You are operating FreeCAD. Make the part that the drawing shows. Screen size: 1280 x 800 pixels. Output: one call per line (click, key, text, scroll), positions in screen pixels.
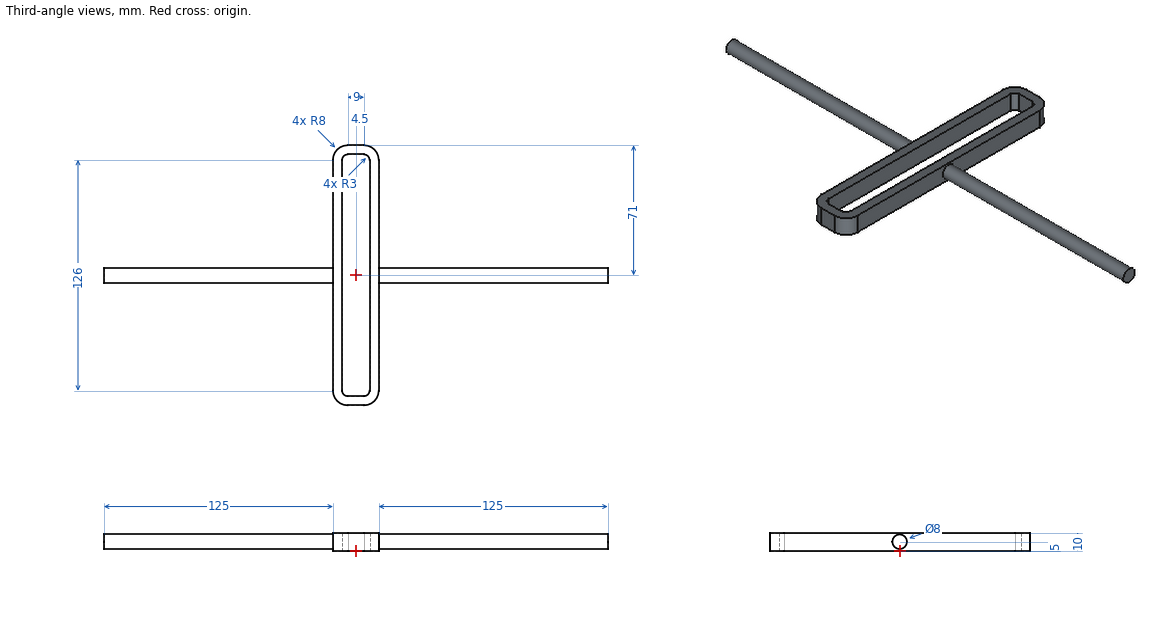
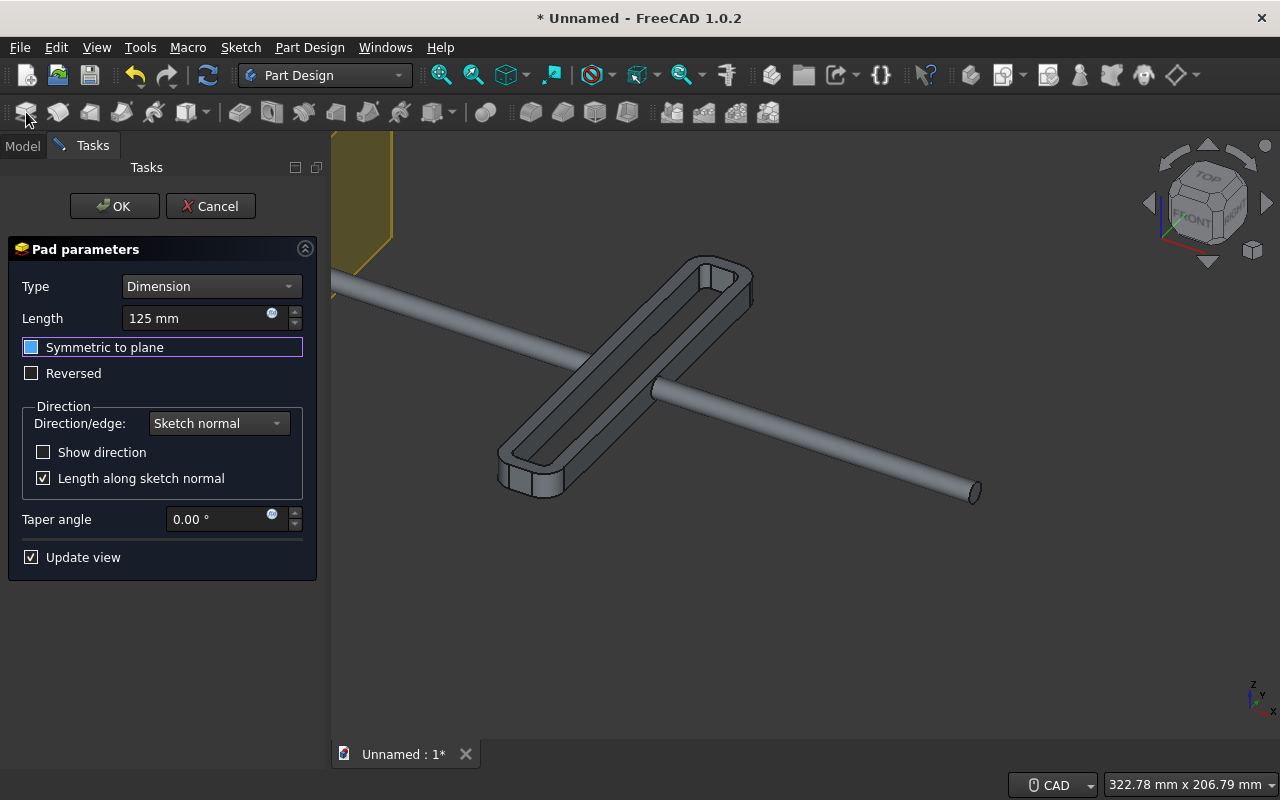
click(115, 206)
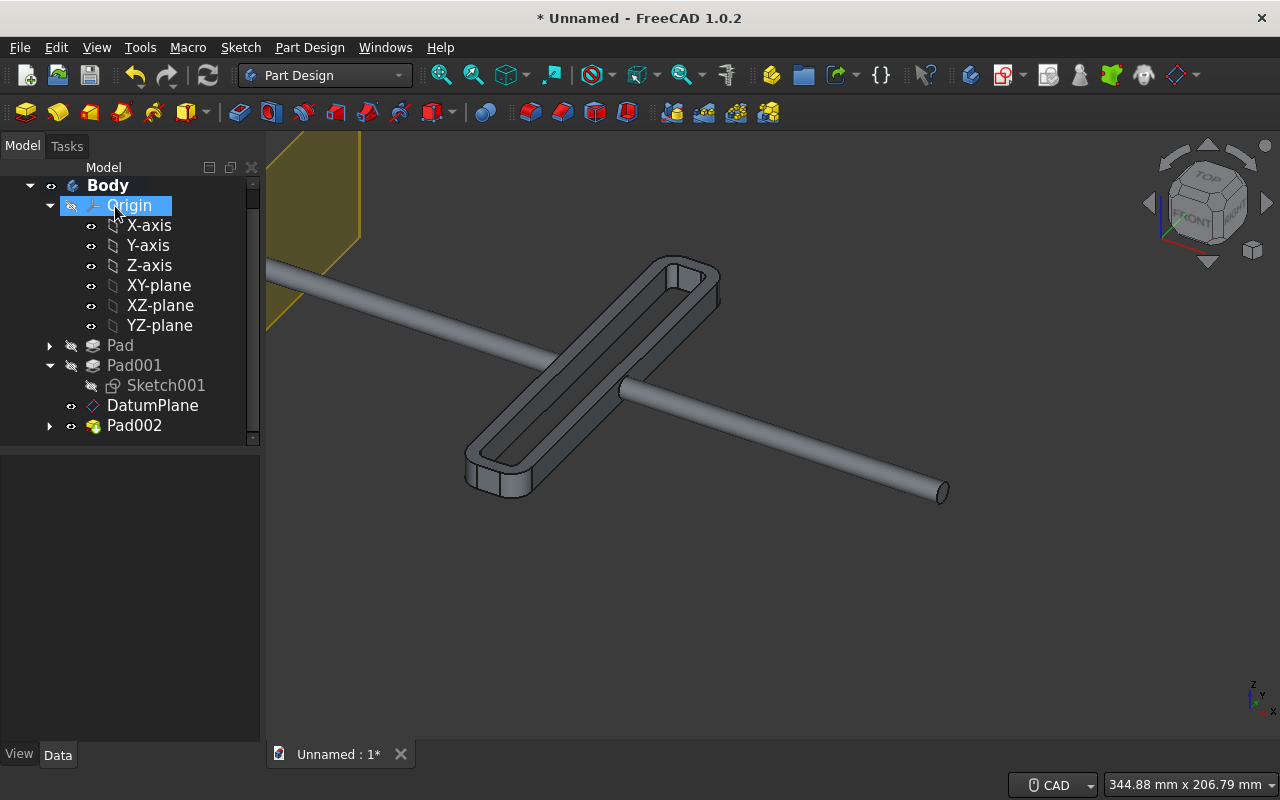
click(116, 406)
key(space)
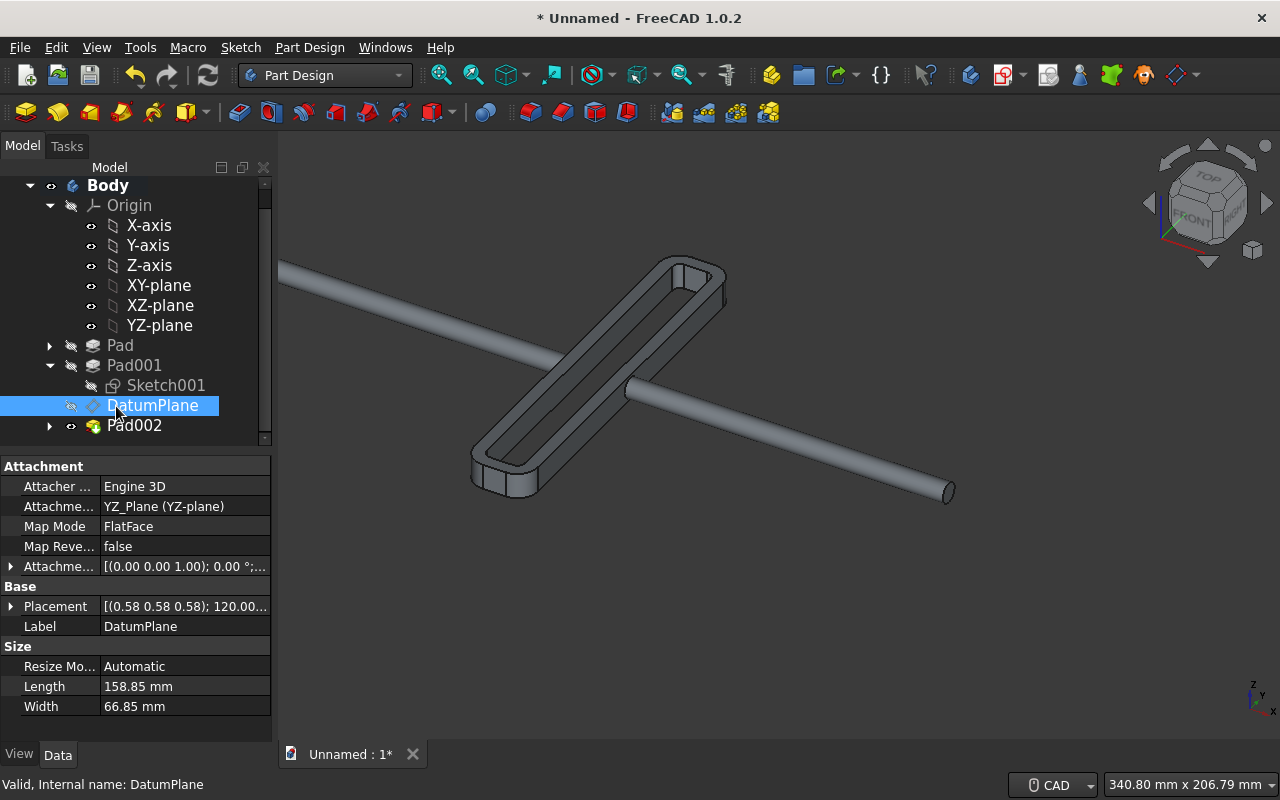
key(0)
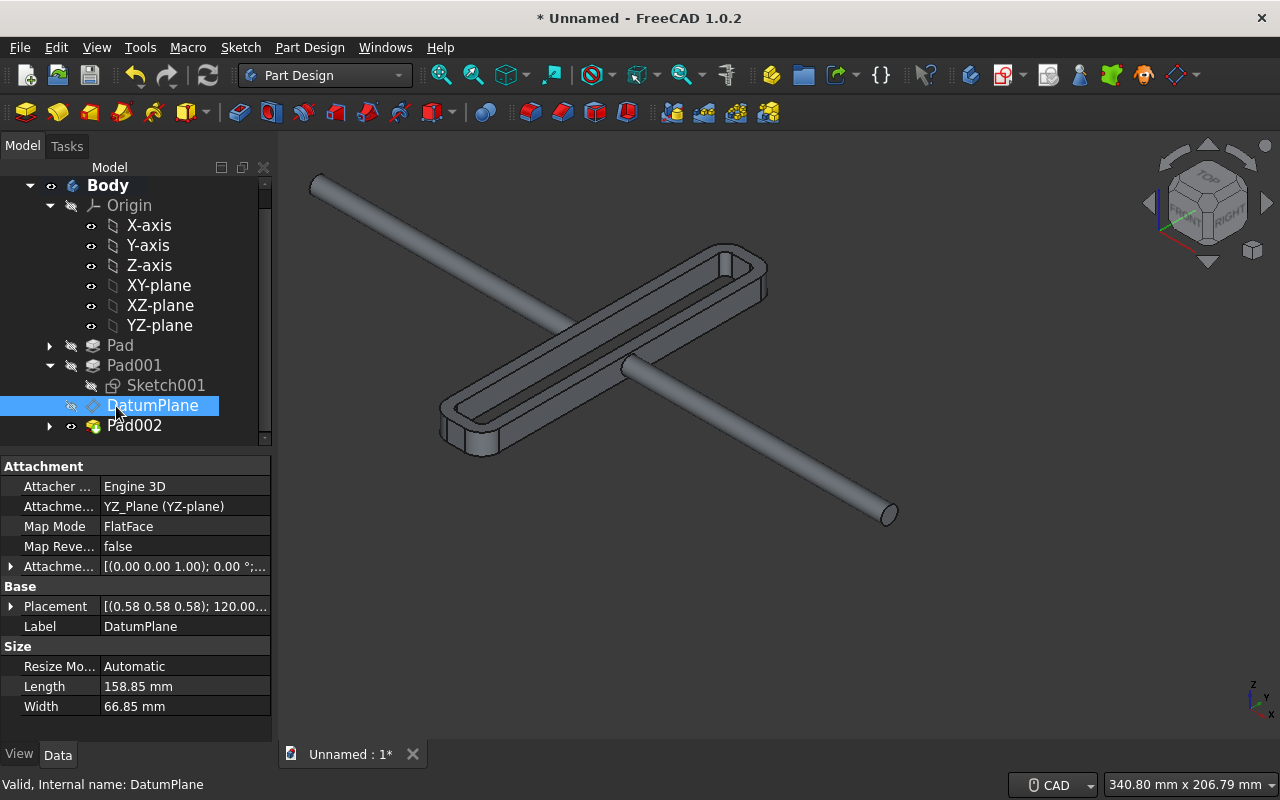
click(442, 76)